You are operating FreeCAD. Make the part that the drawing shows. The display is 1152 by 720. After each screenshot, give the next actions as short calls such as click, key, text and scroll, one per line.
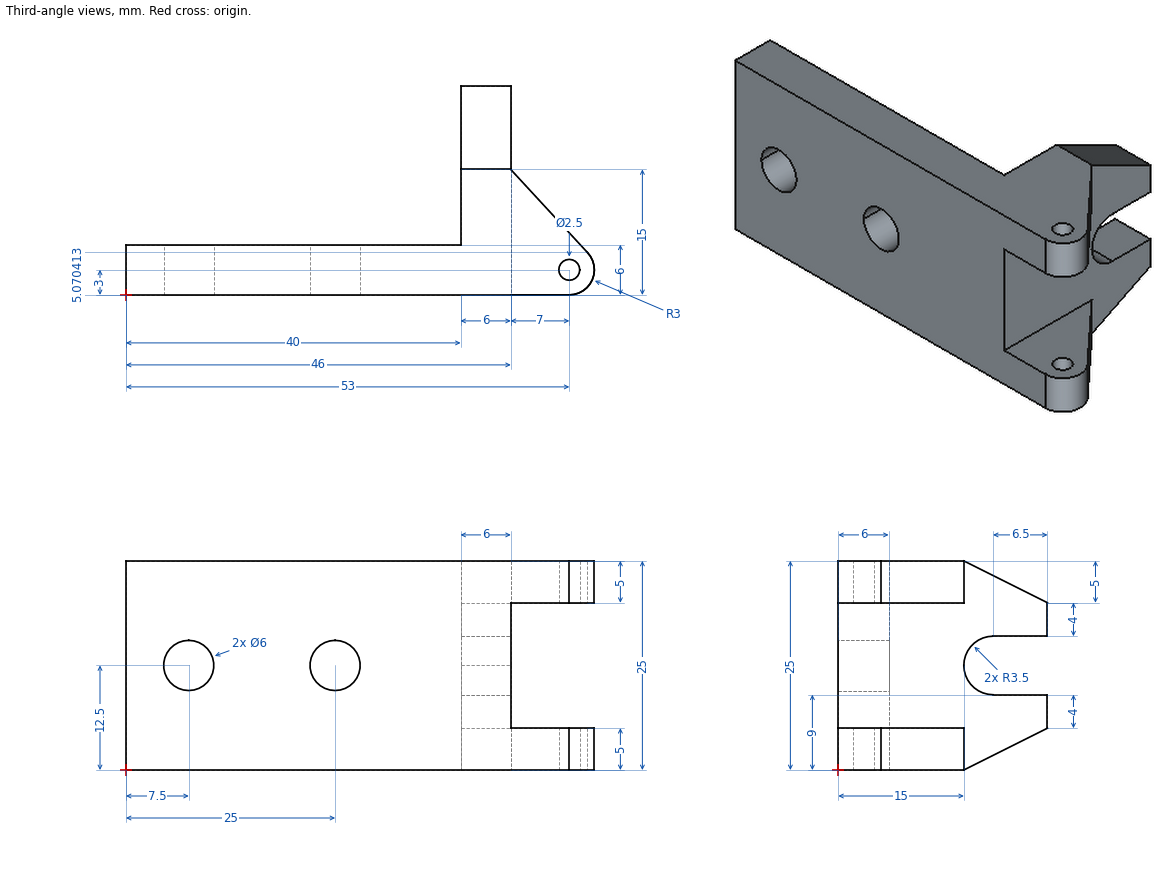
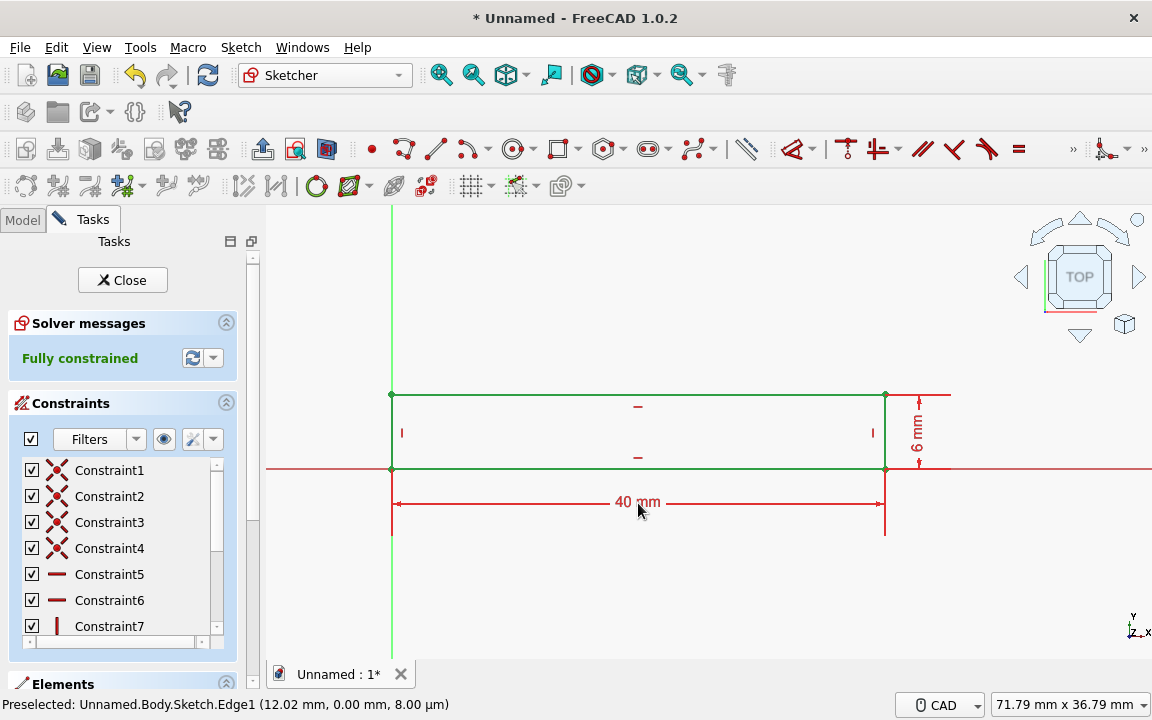
click(123, 280)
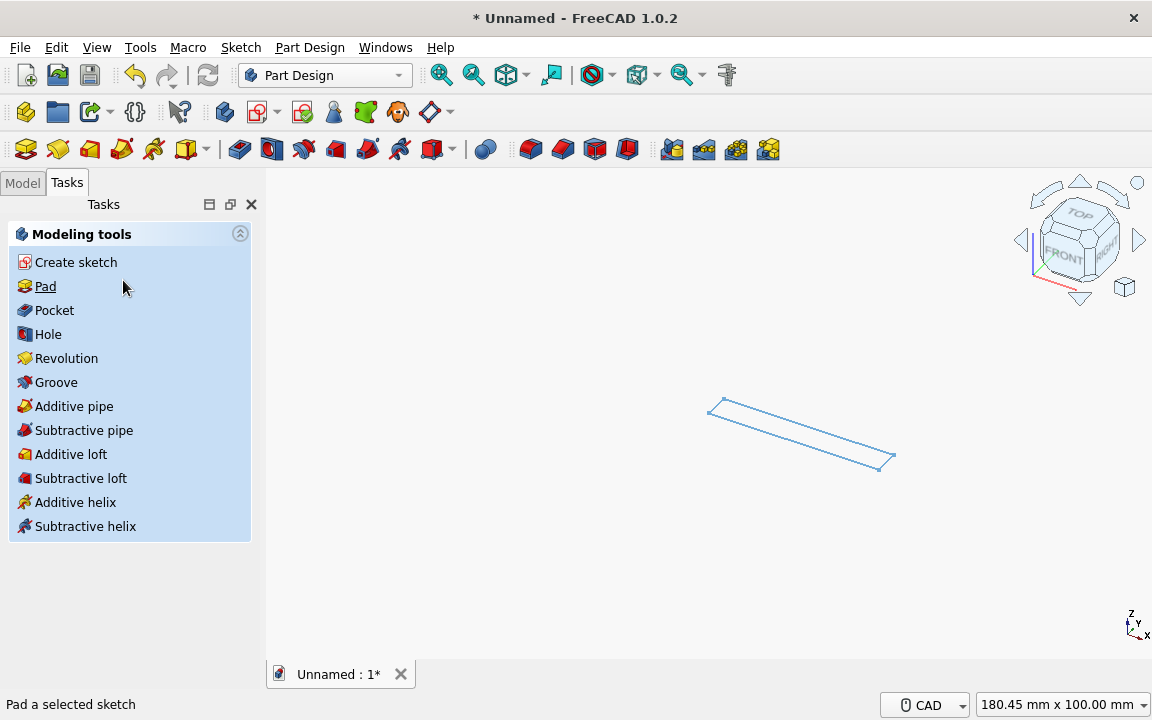
click(26, 150)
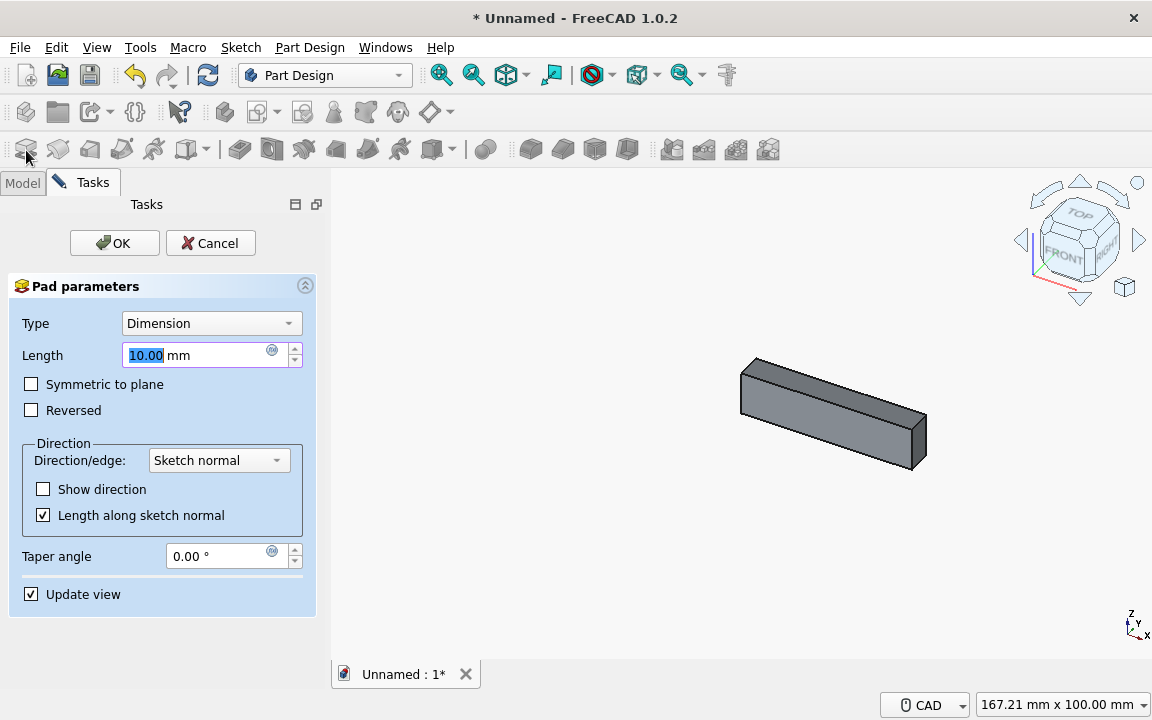
text(25)
key(Tab)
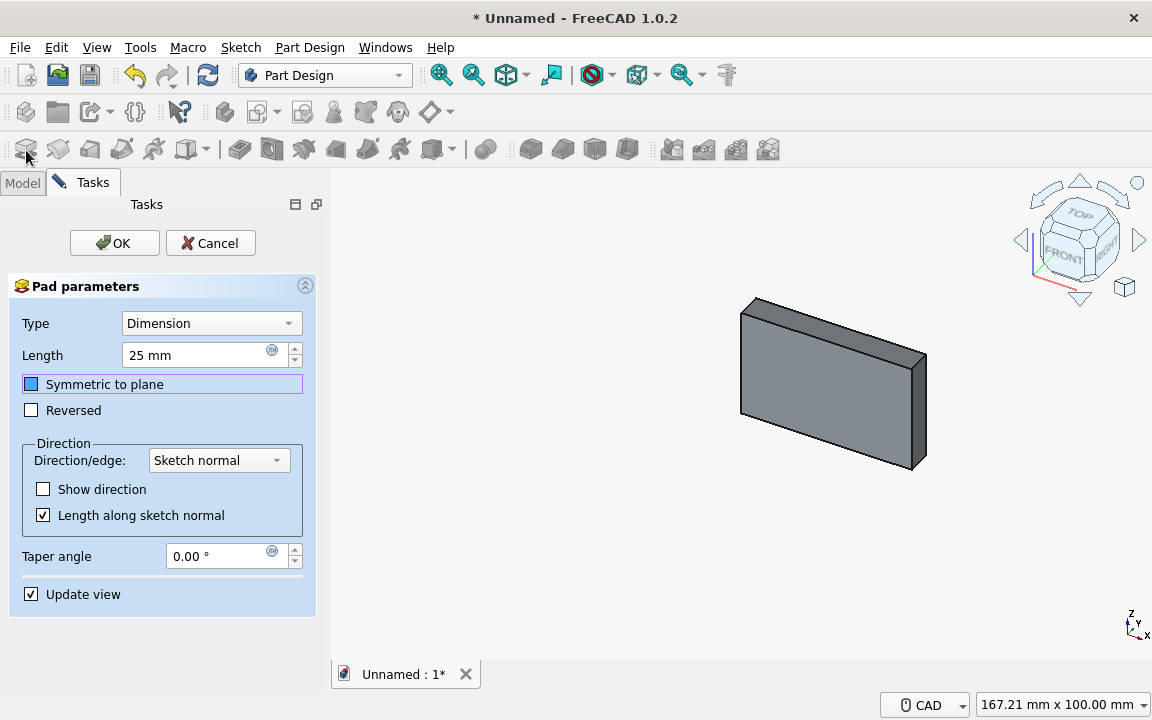
click(115, 243)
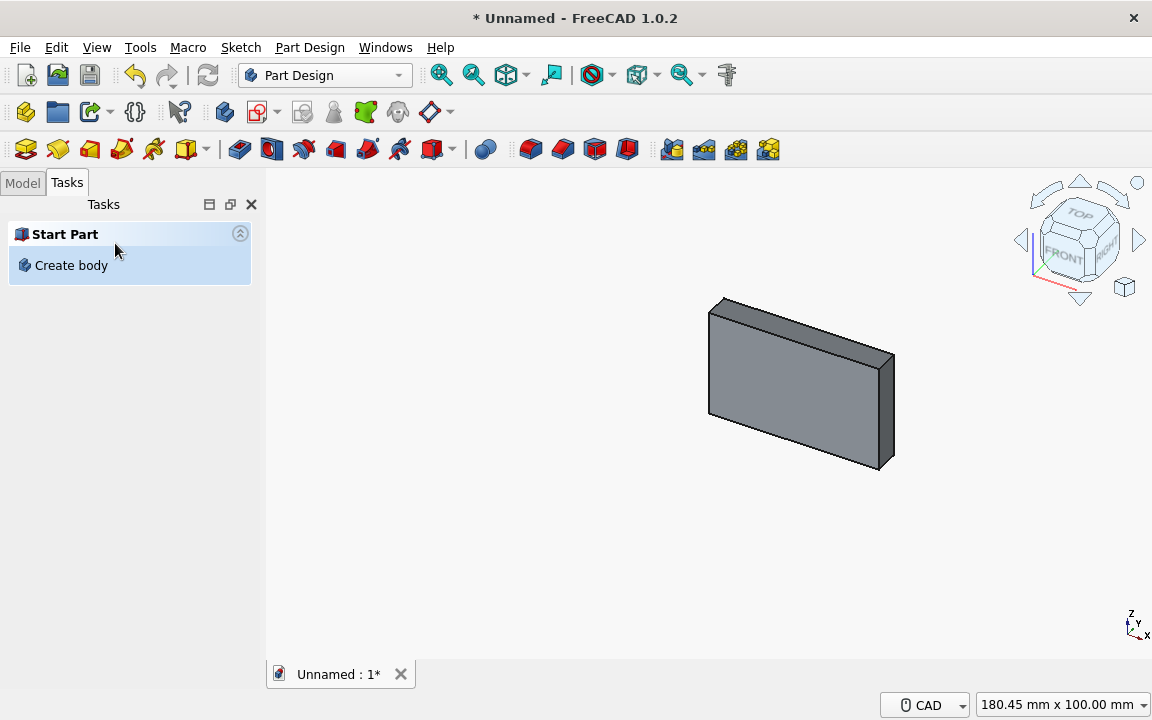
key(v)
key(f)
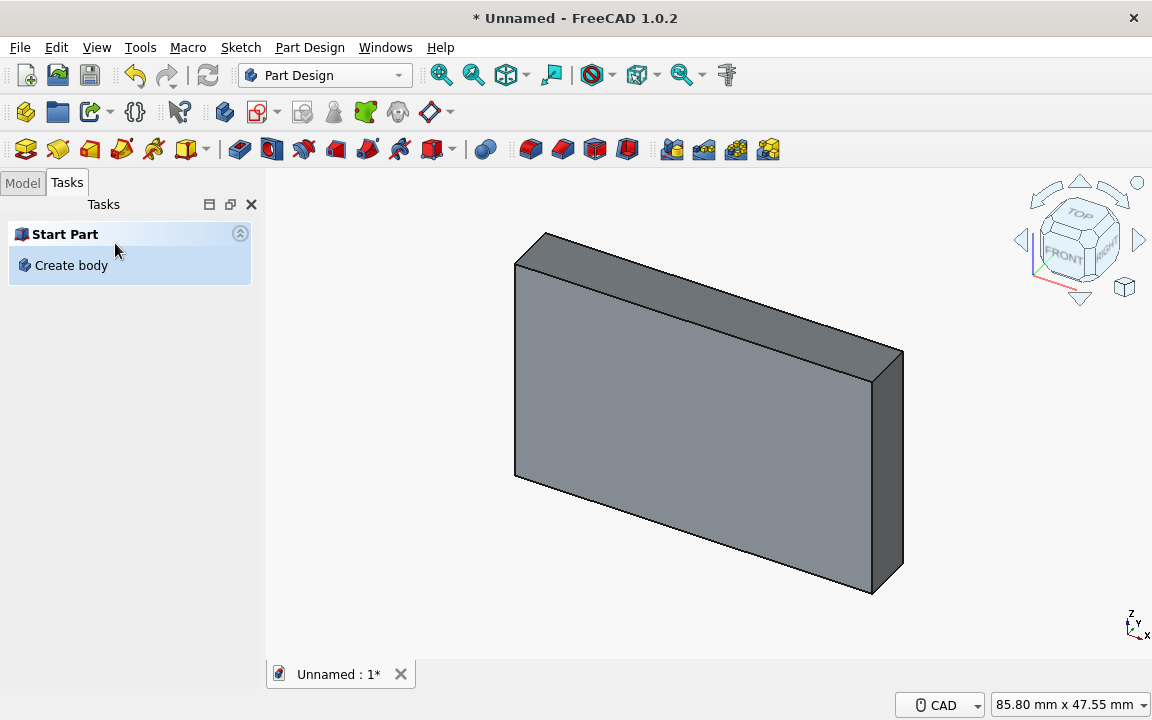
click(811, 341)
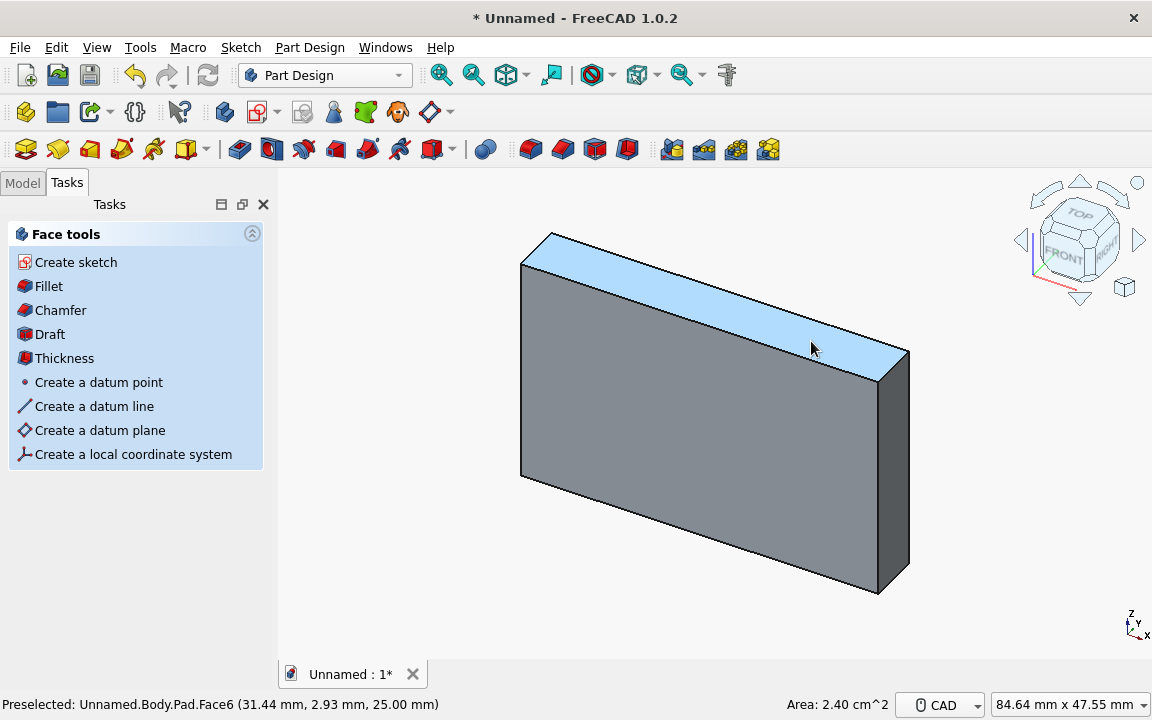
click(258, 112)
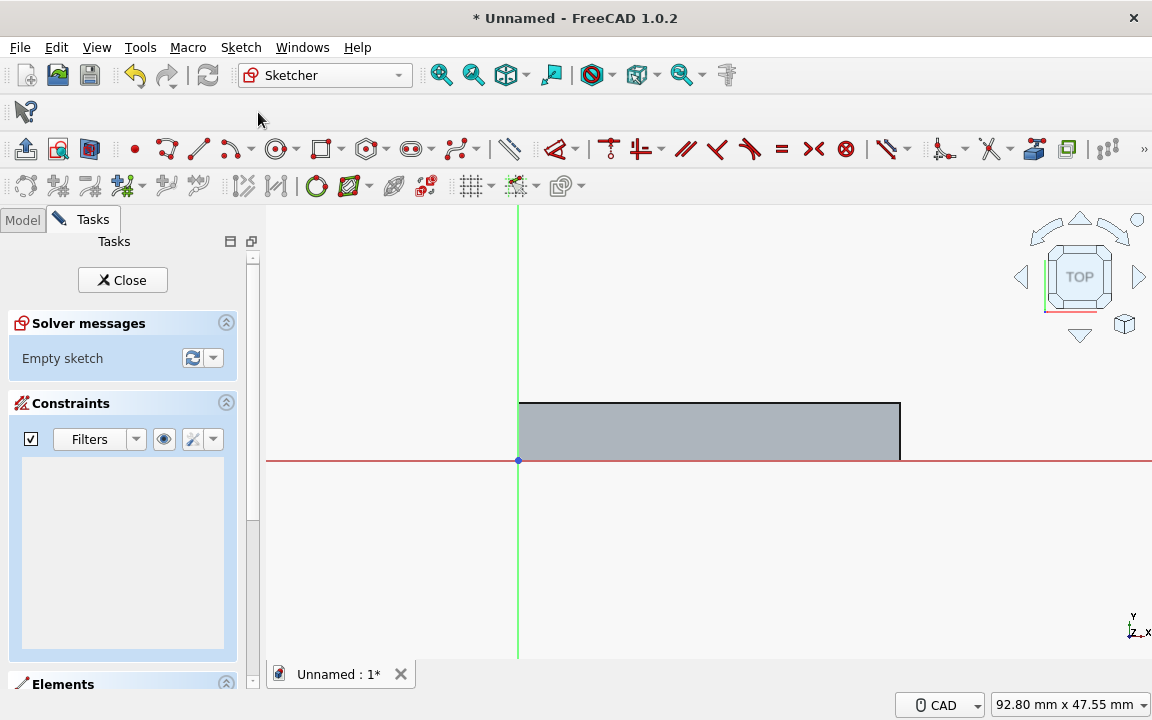
scroll(987, 337, up, 3)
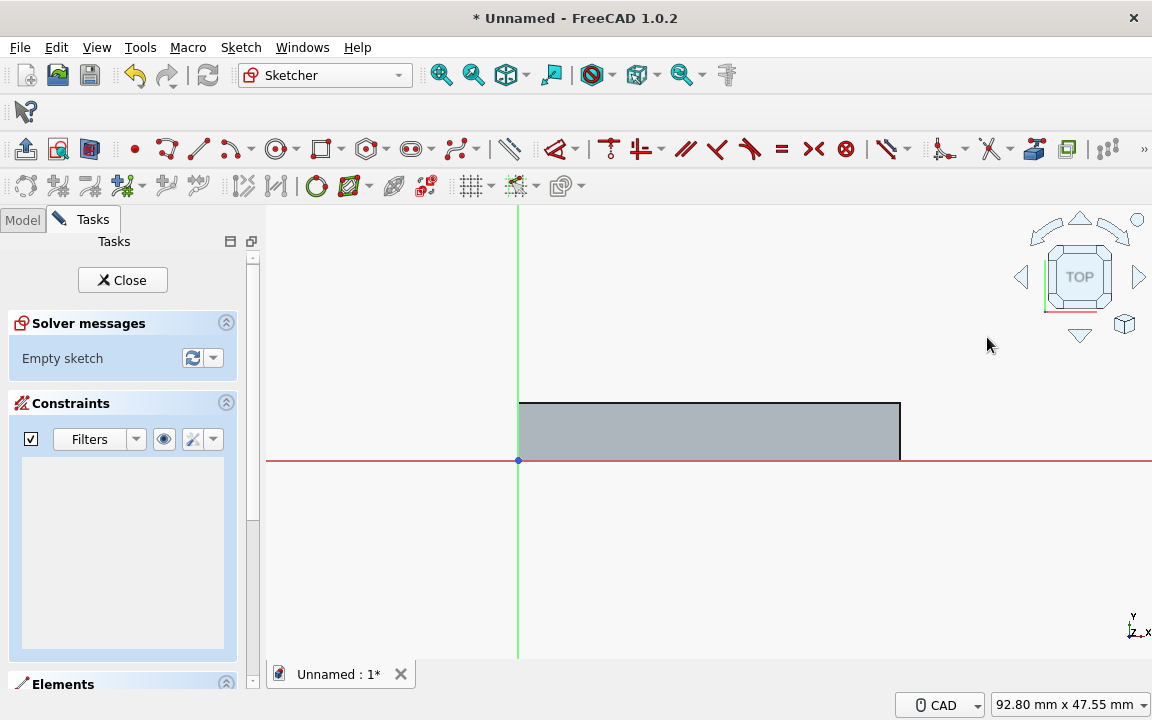
click(322, 150)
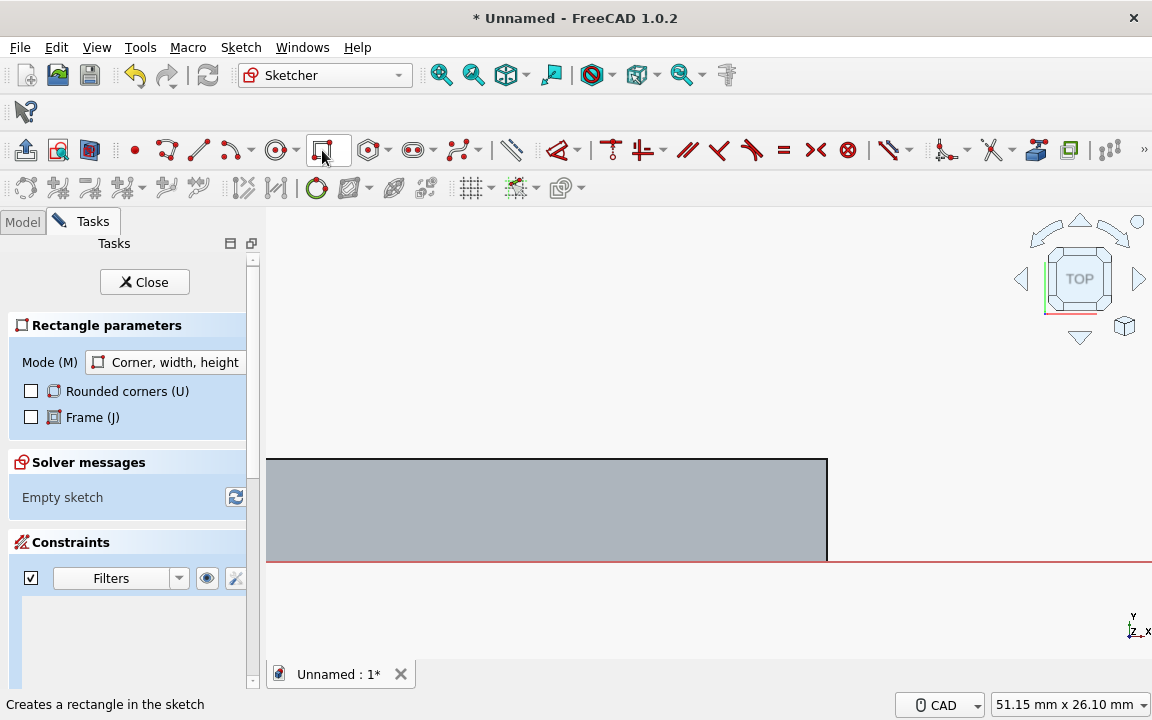
click(827, 303)
click(931, 562)
key(Escape)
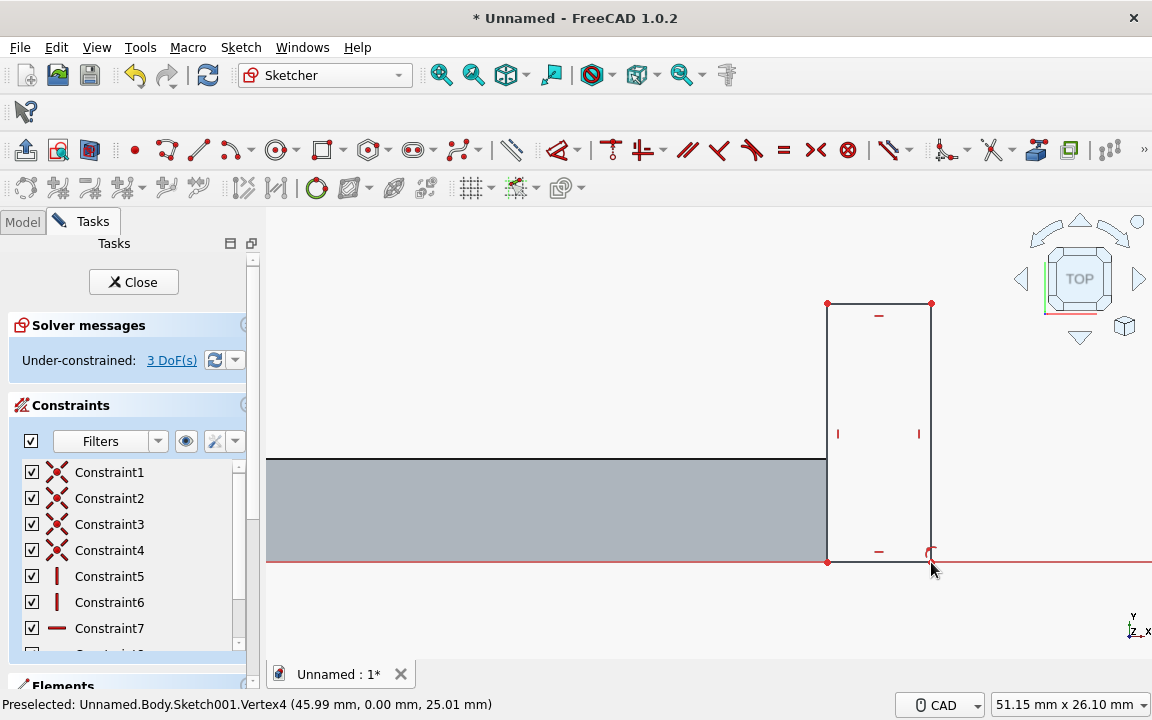
key(d)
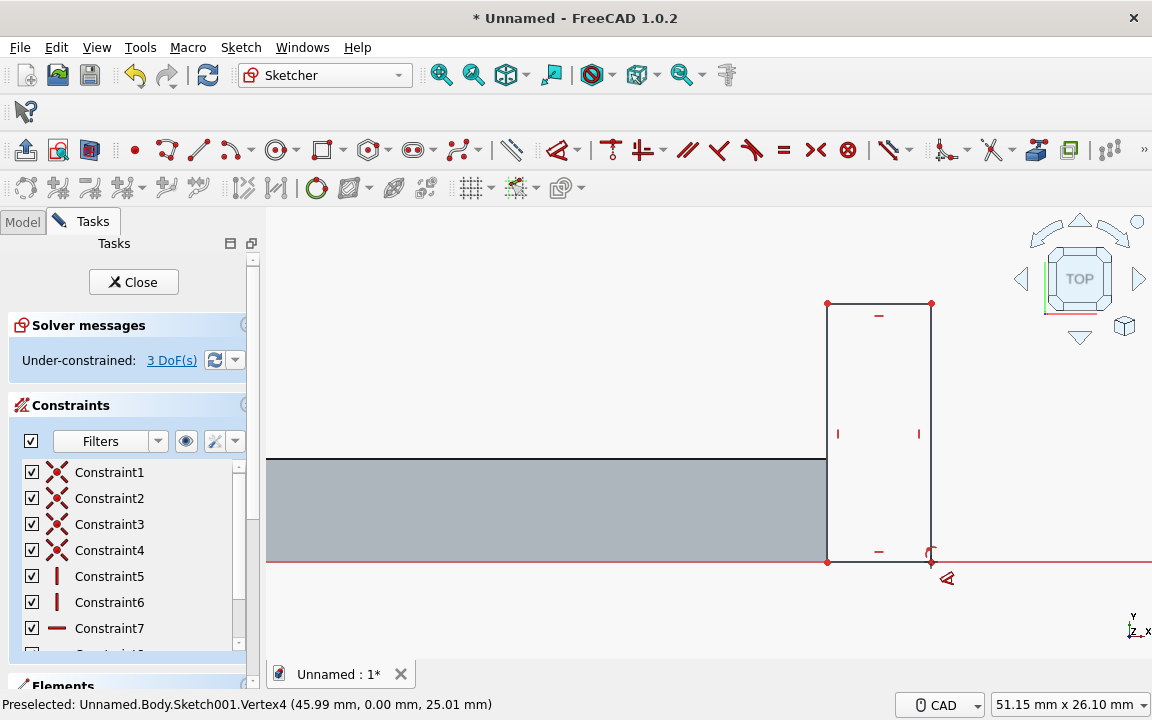
click(858, 562)
click(879, 596)